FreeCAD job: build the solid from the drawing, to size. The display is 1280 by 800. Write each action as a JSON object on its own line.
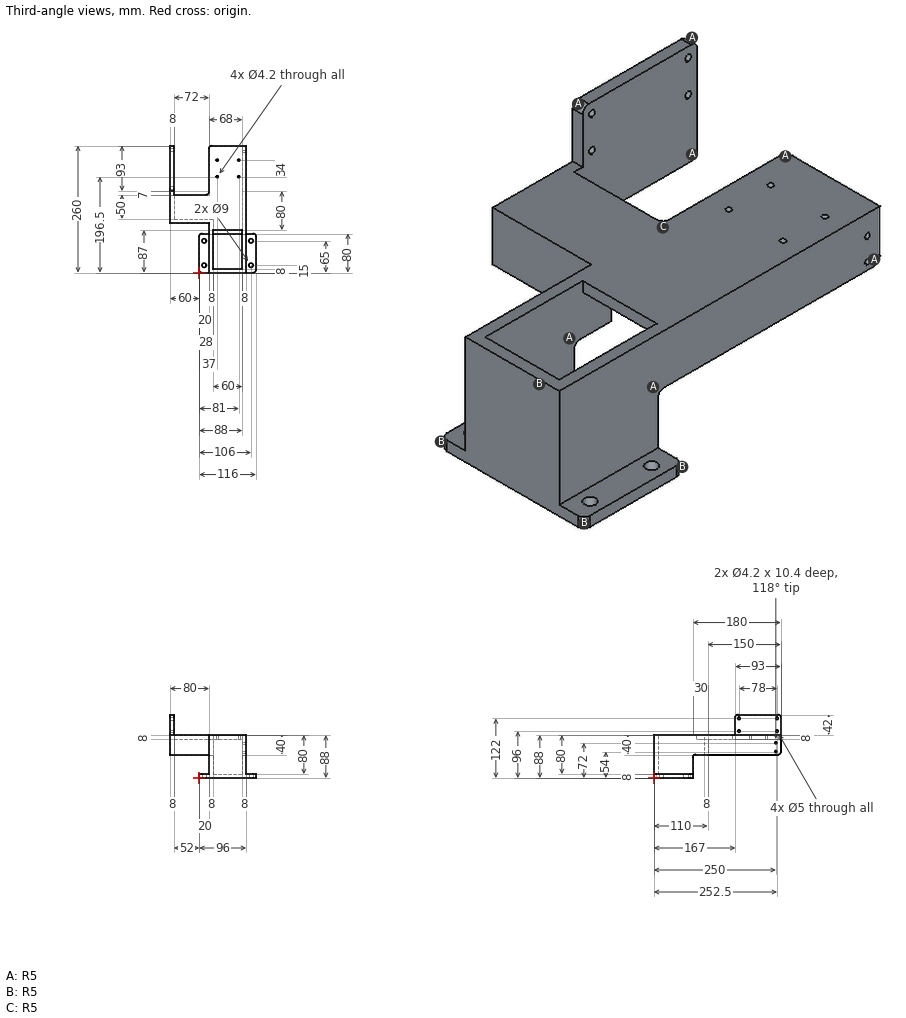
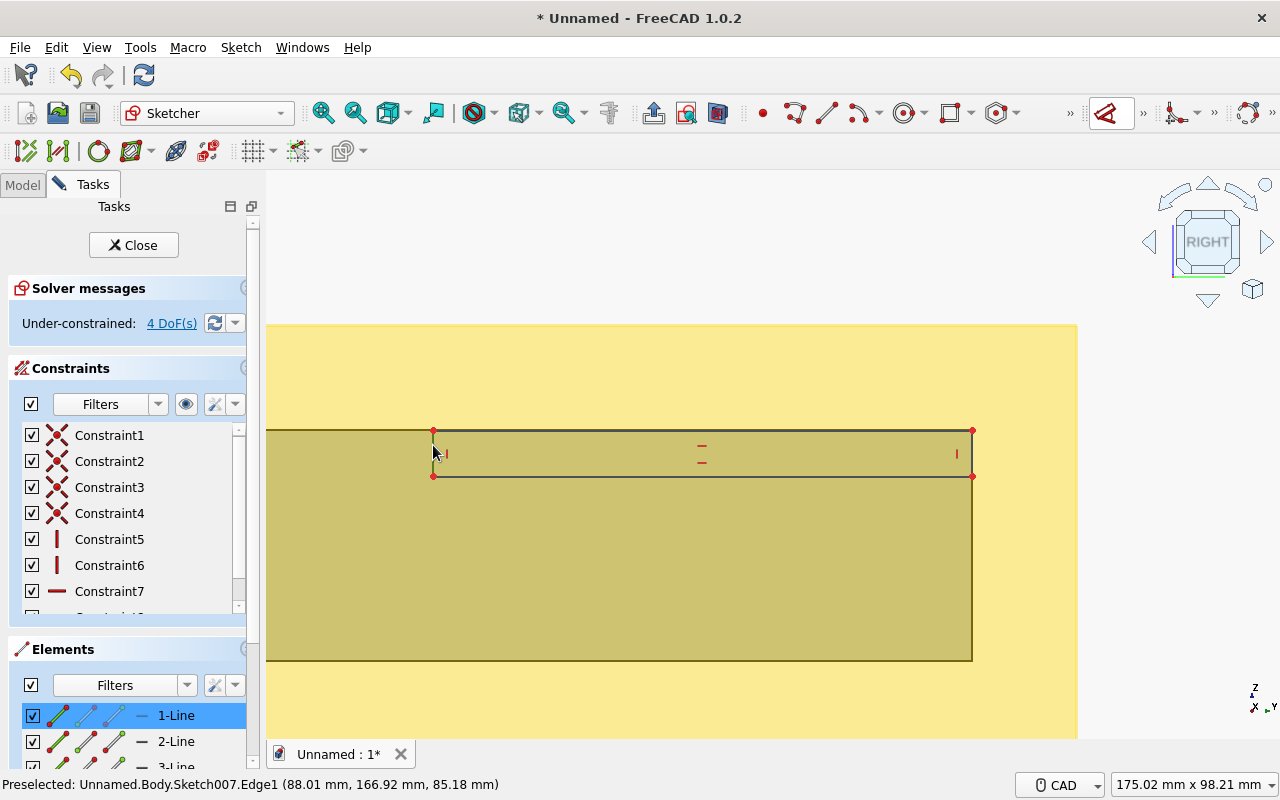
{"action": "left_click", "coordinate": [1128, 114]}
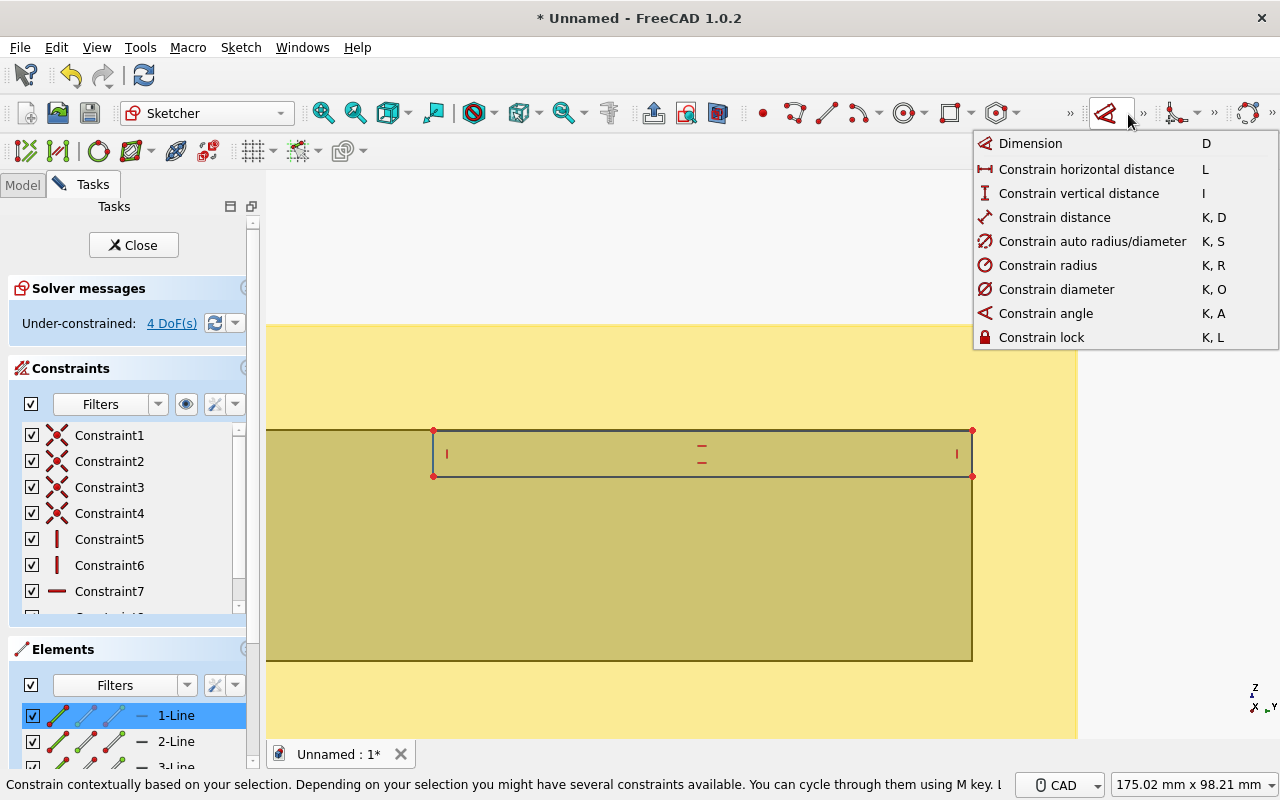
{"action": "left_click", "coordinate": [1126, 193]}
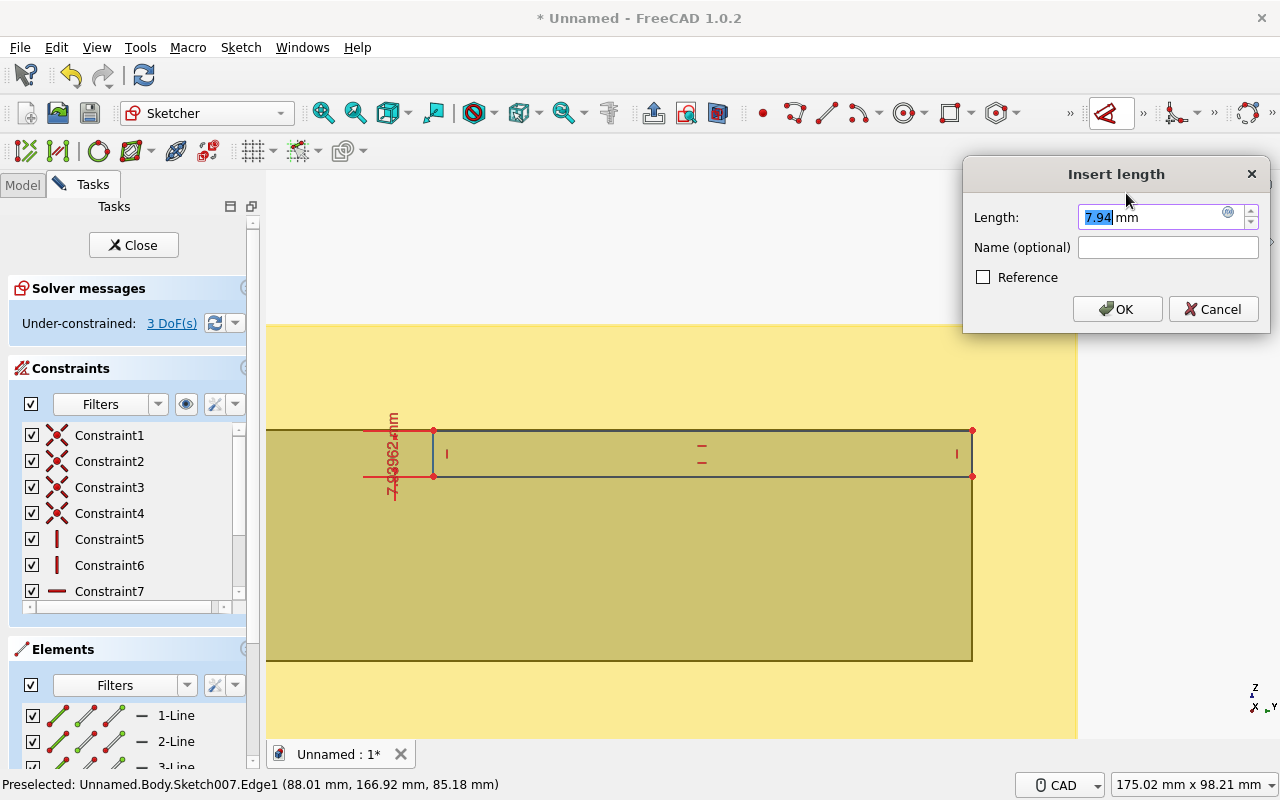
{"action": "type", "text": "8"}
{"action": "key", "text": "Return"}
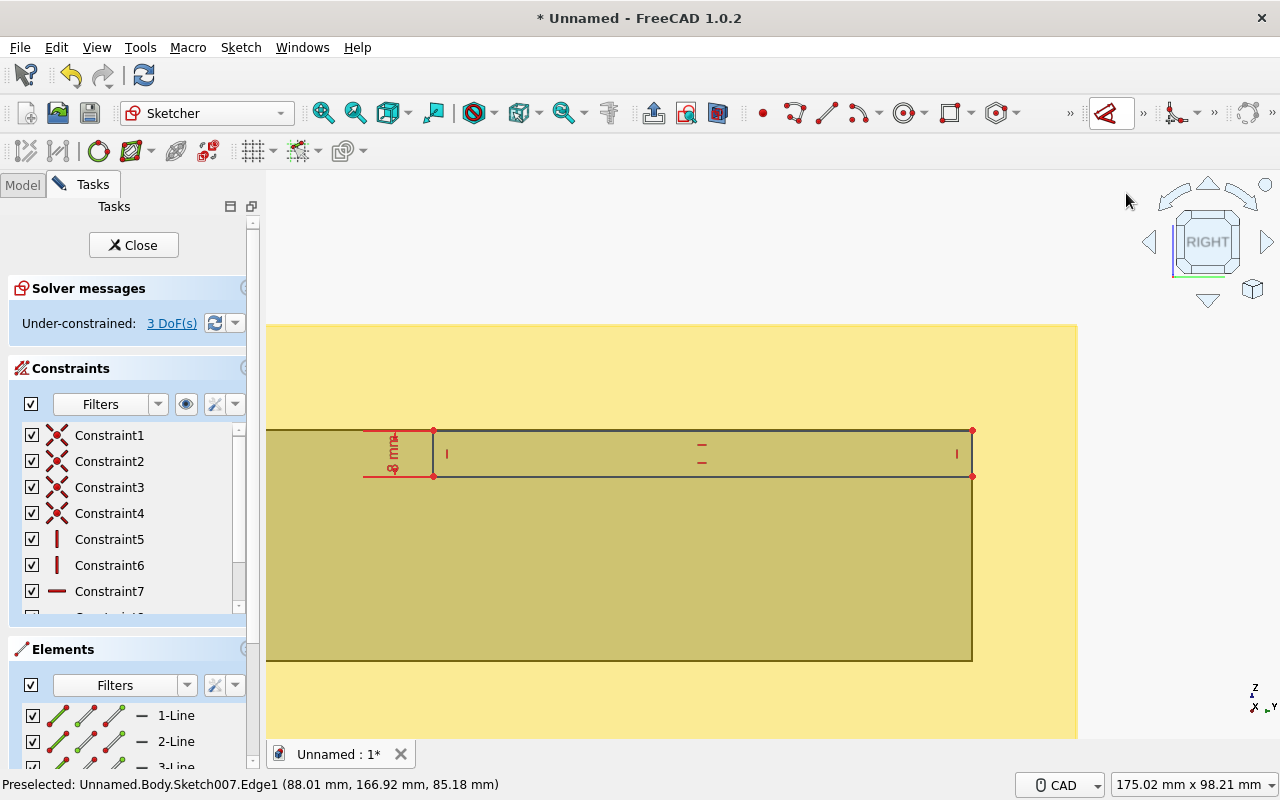
{"action": "left_click", "coordinate": [595, 477]}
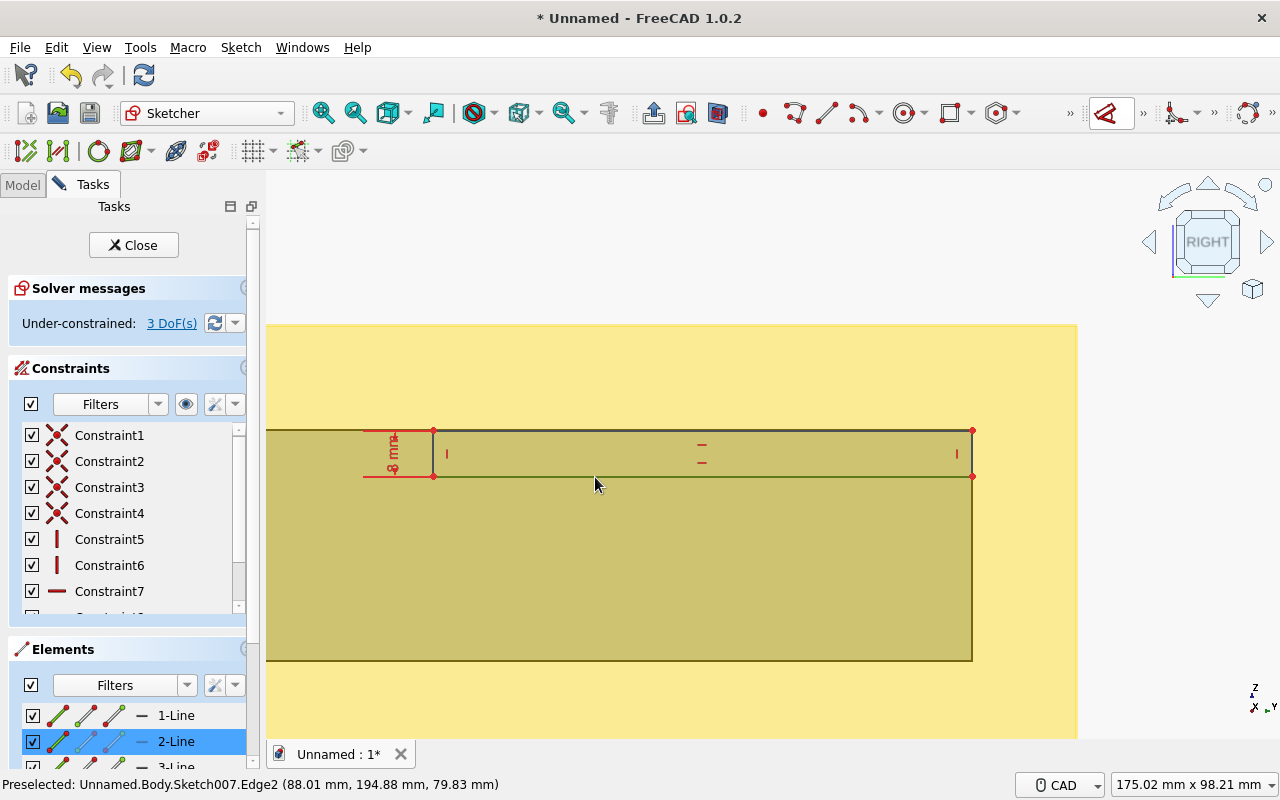
{"action": "left_click", "coordinate": [1128, 114]}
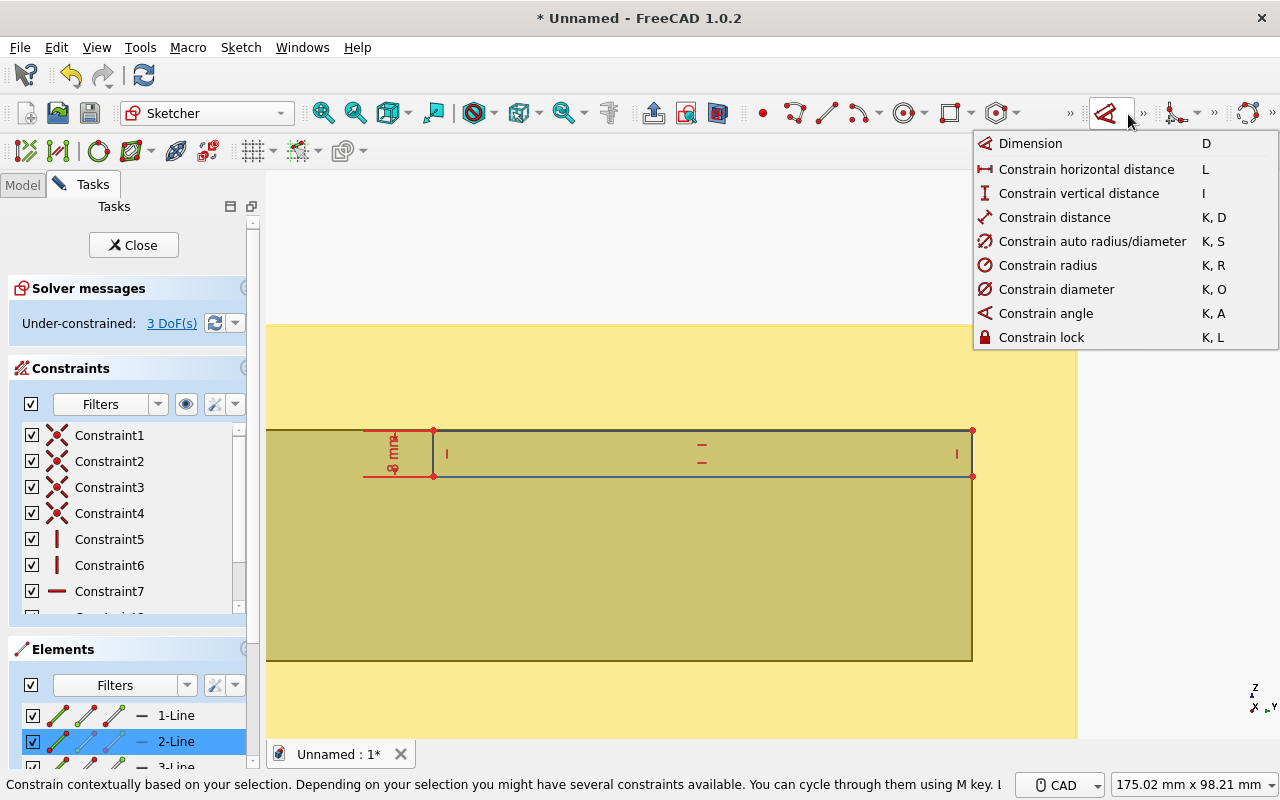
{"action": "left_click", "coordinate": [1126, 169]}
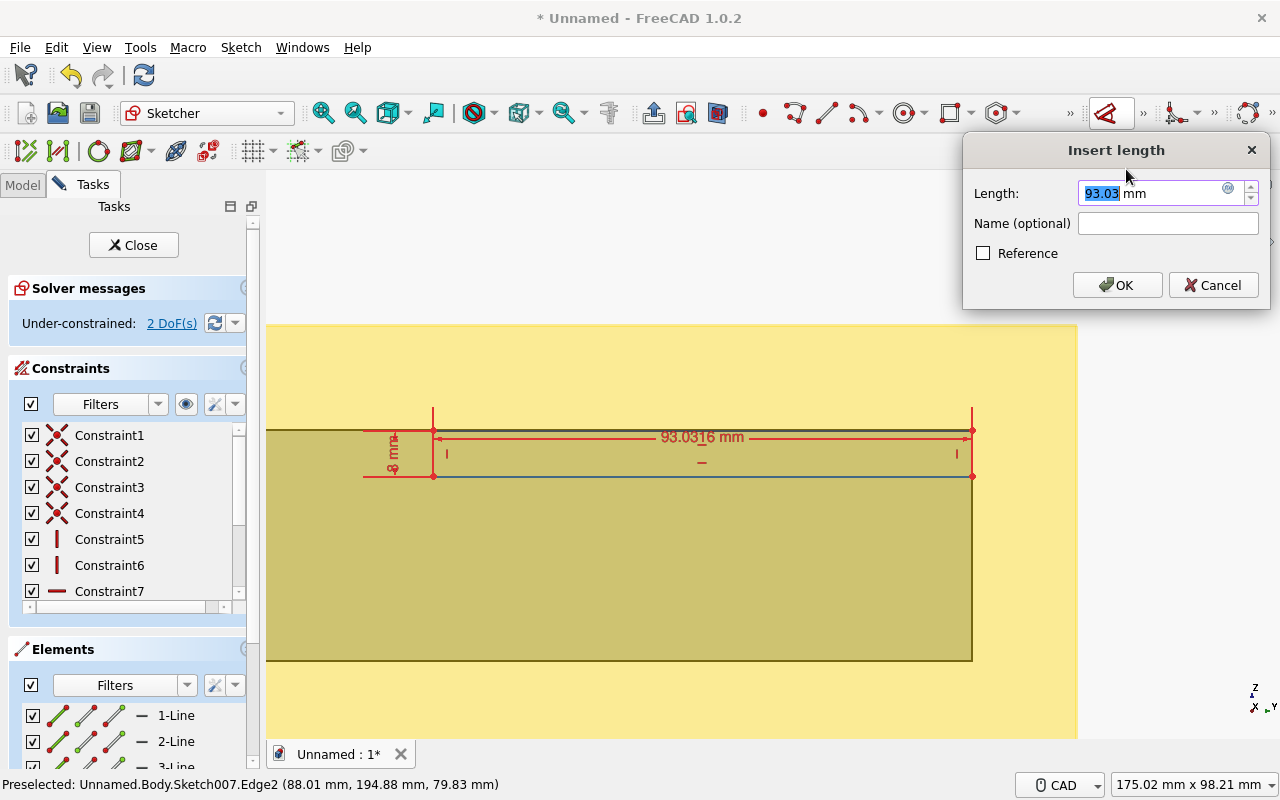
{"action": "type", "text": "93"}
{"action": "key", "text": "Return"}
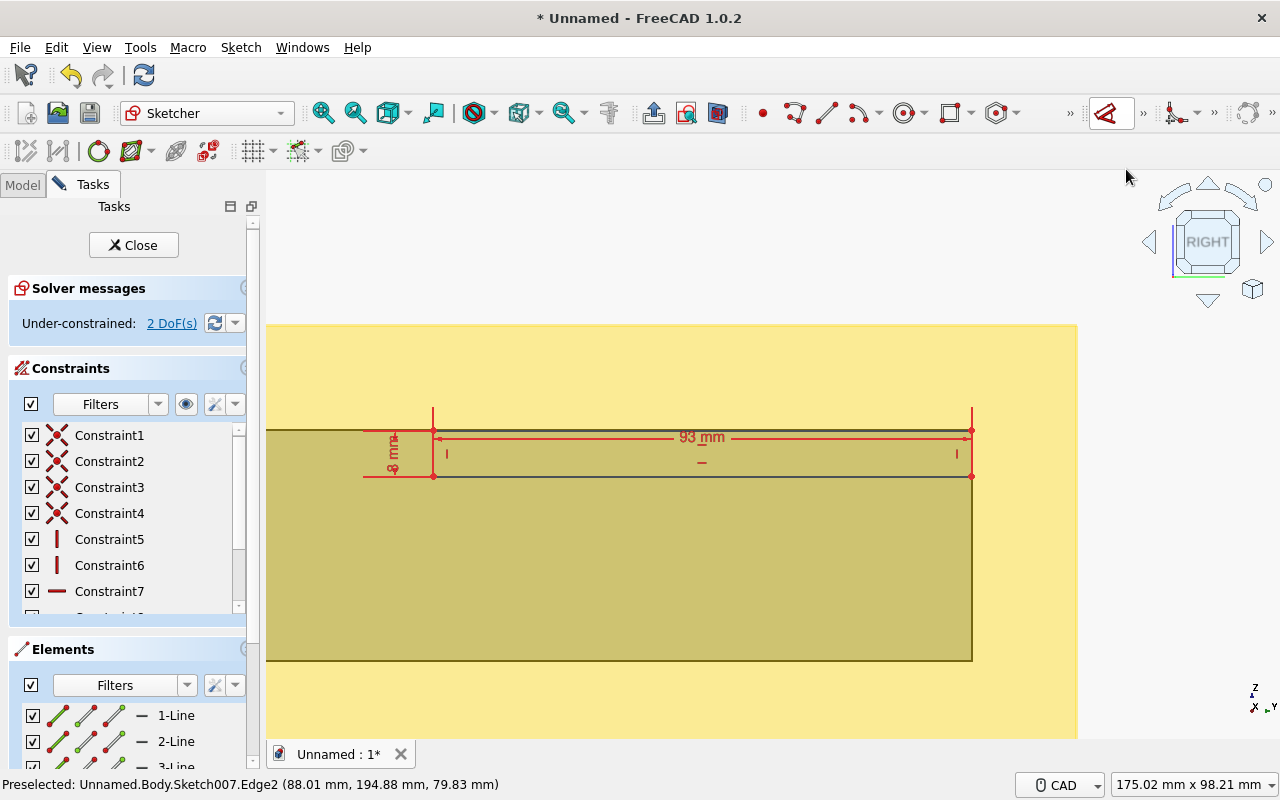
{"action": "left_click", "coordinate": [433, 431]}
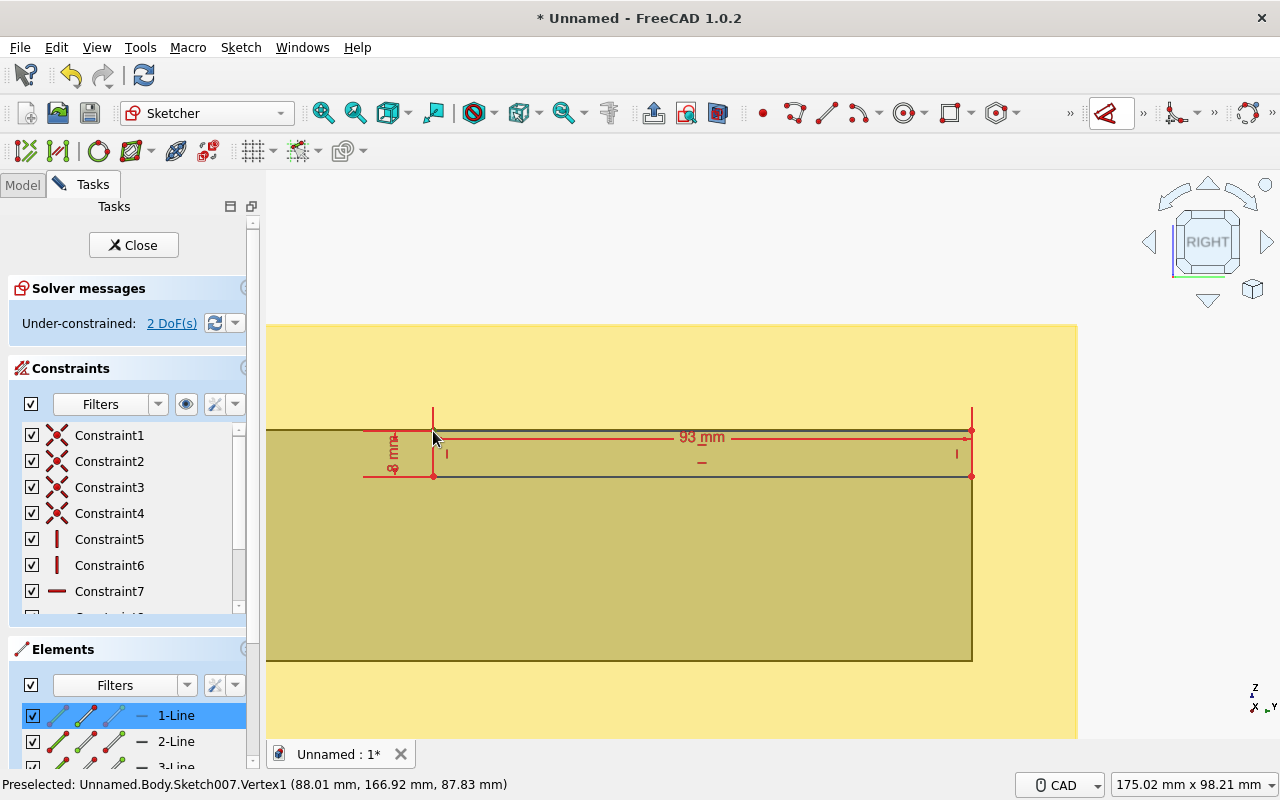
{"action": "key", "text": "i"}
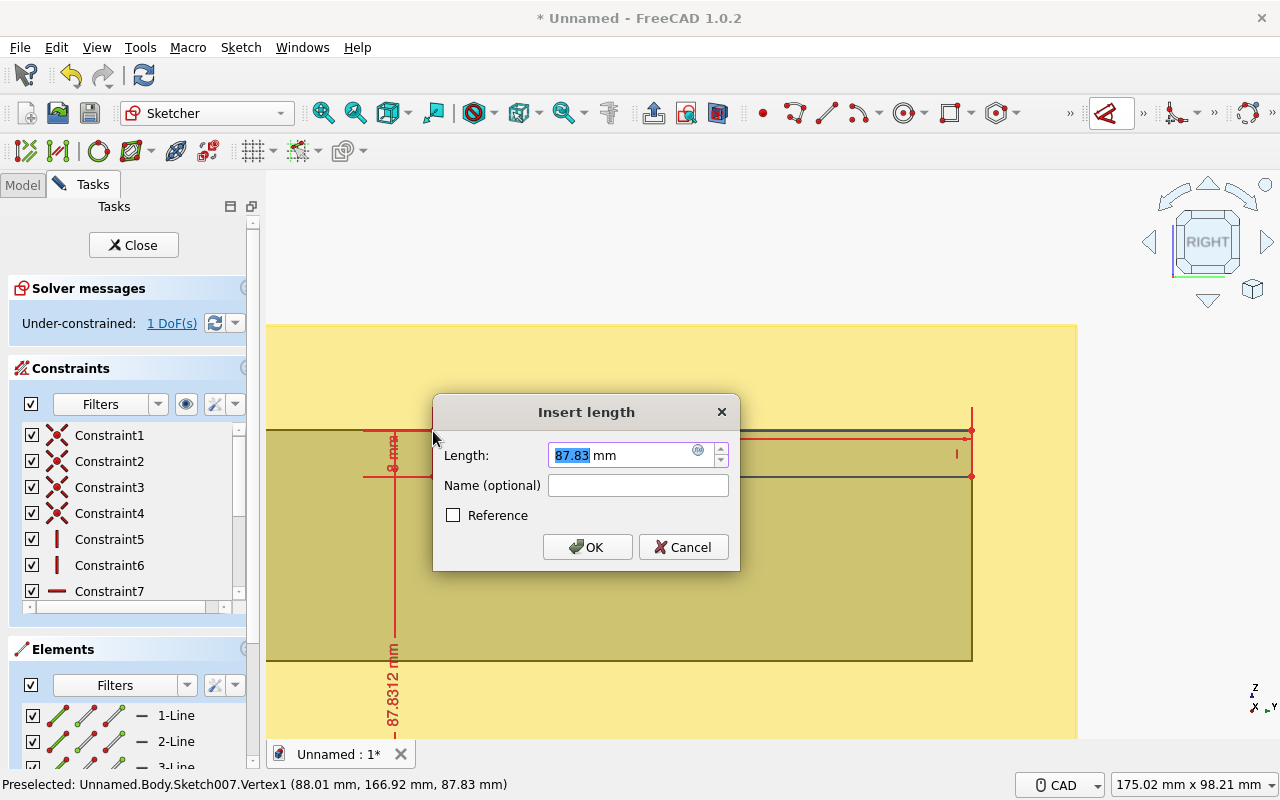
{"action": "type", "text": "88"}
{"action": "key", "text": "Return"}